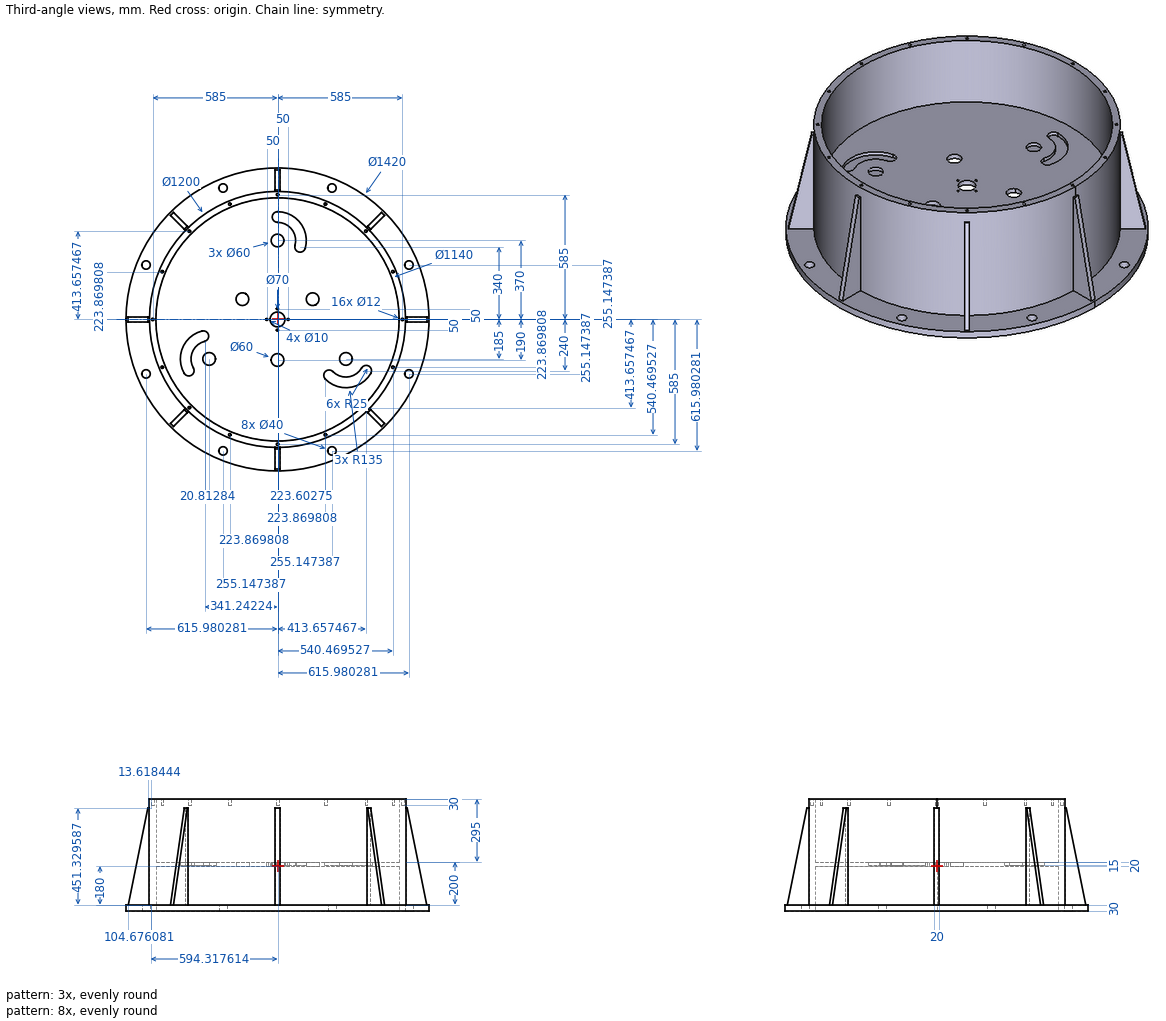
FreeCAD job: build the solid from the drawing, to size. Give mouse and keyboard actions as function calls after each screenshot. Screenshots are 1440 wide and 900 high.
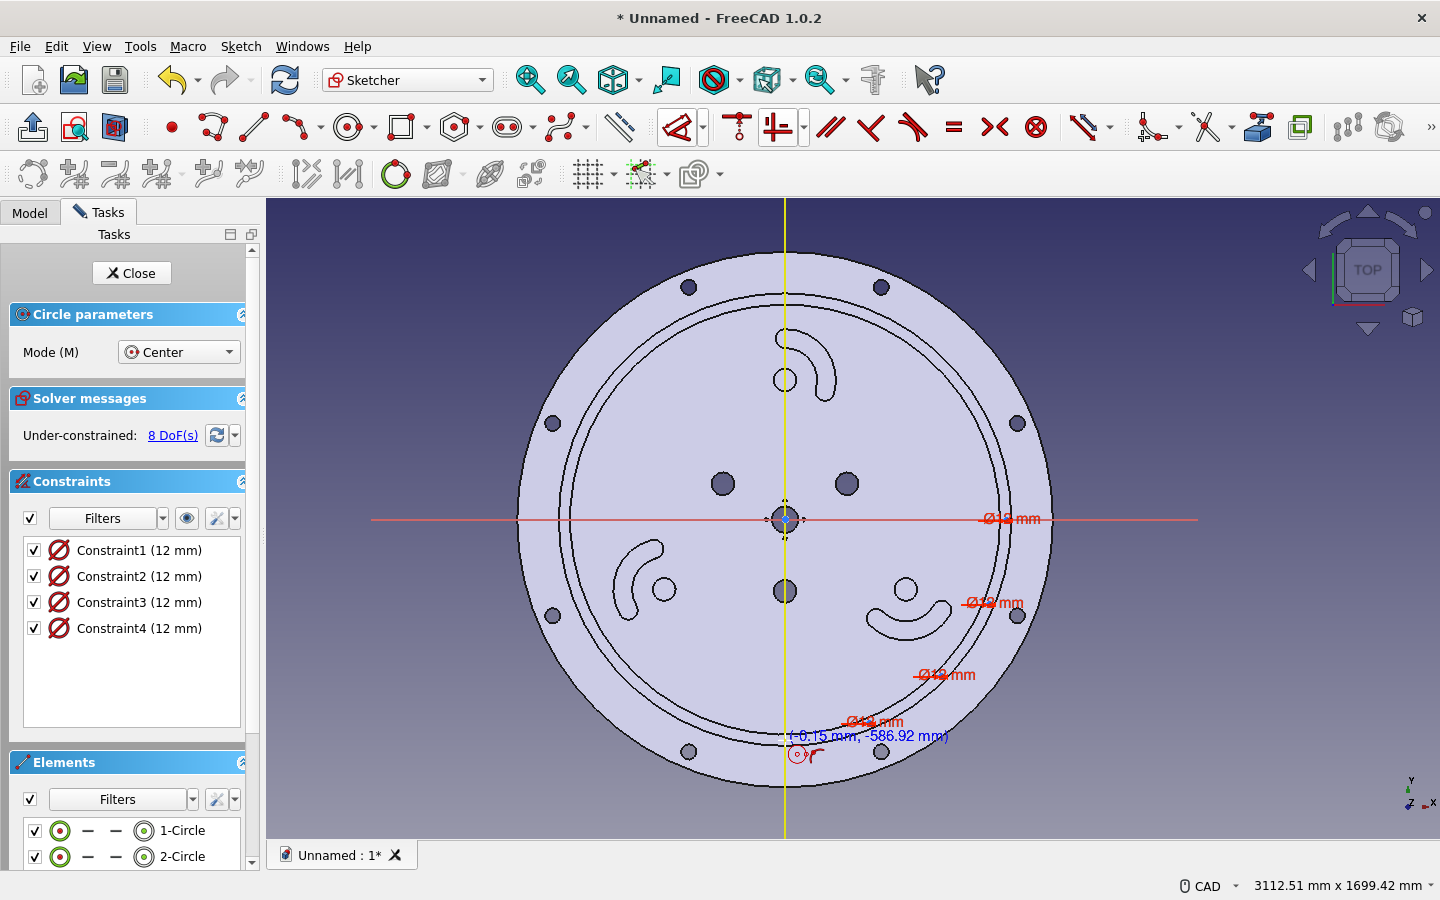
click(785, 740)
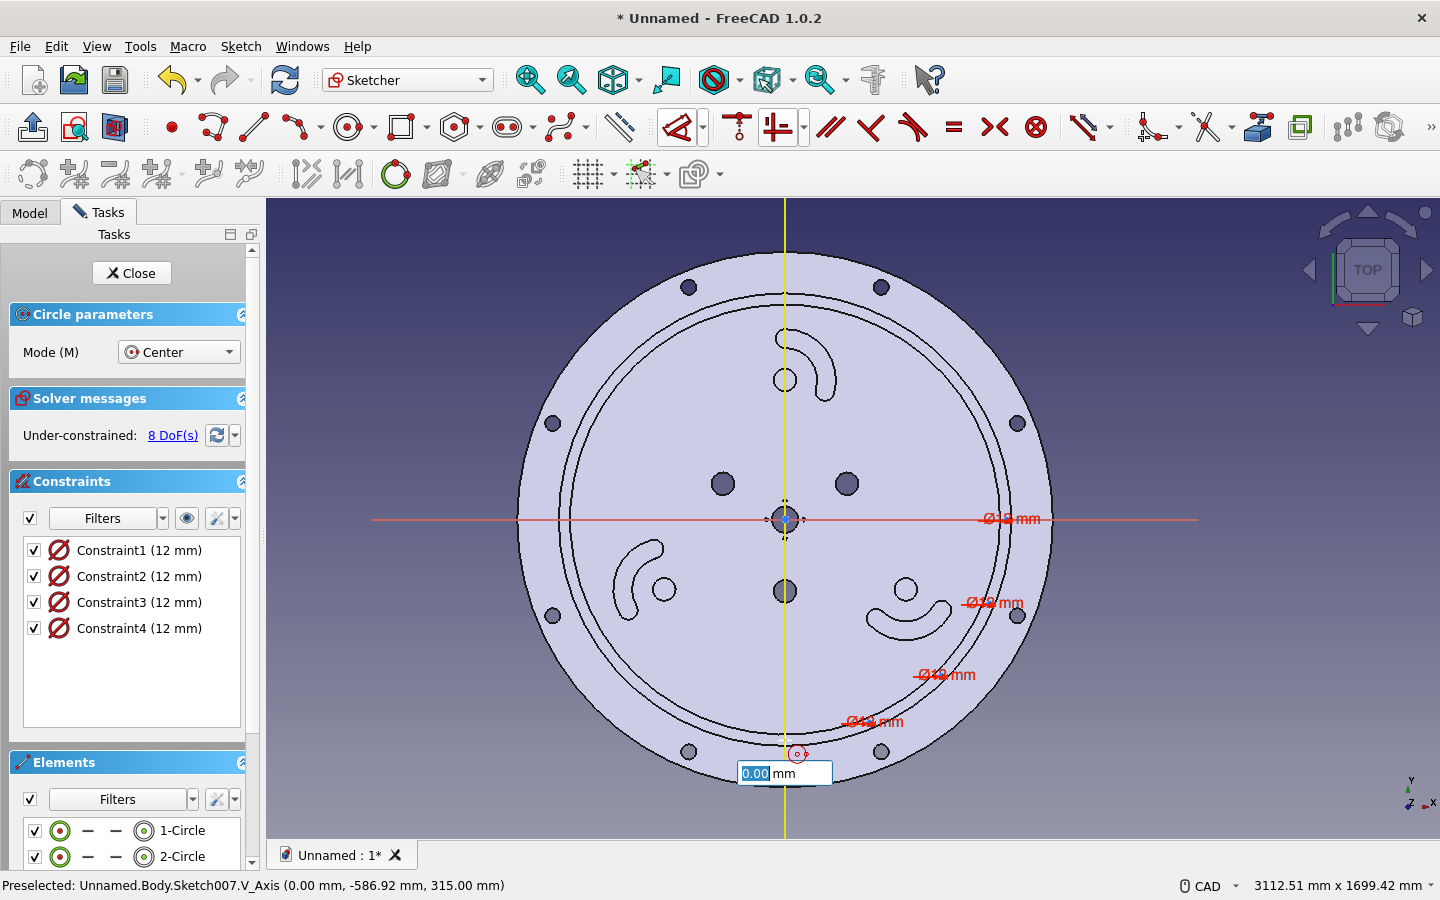
scroll(787, 740, up, 11)
move(785, 729)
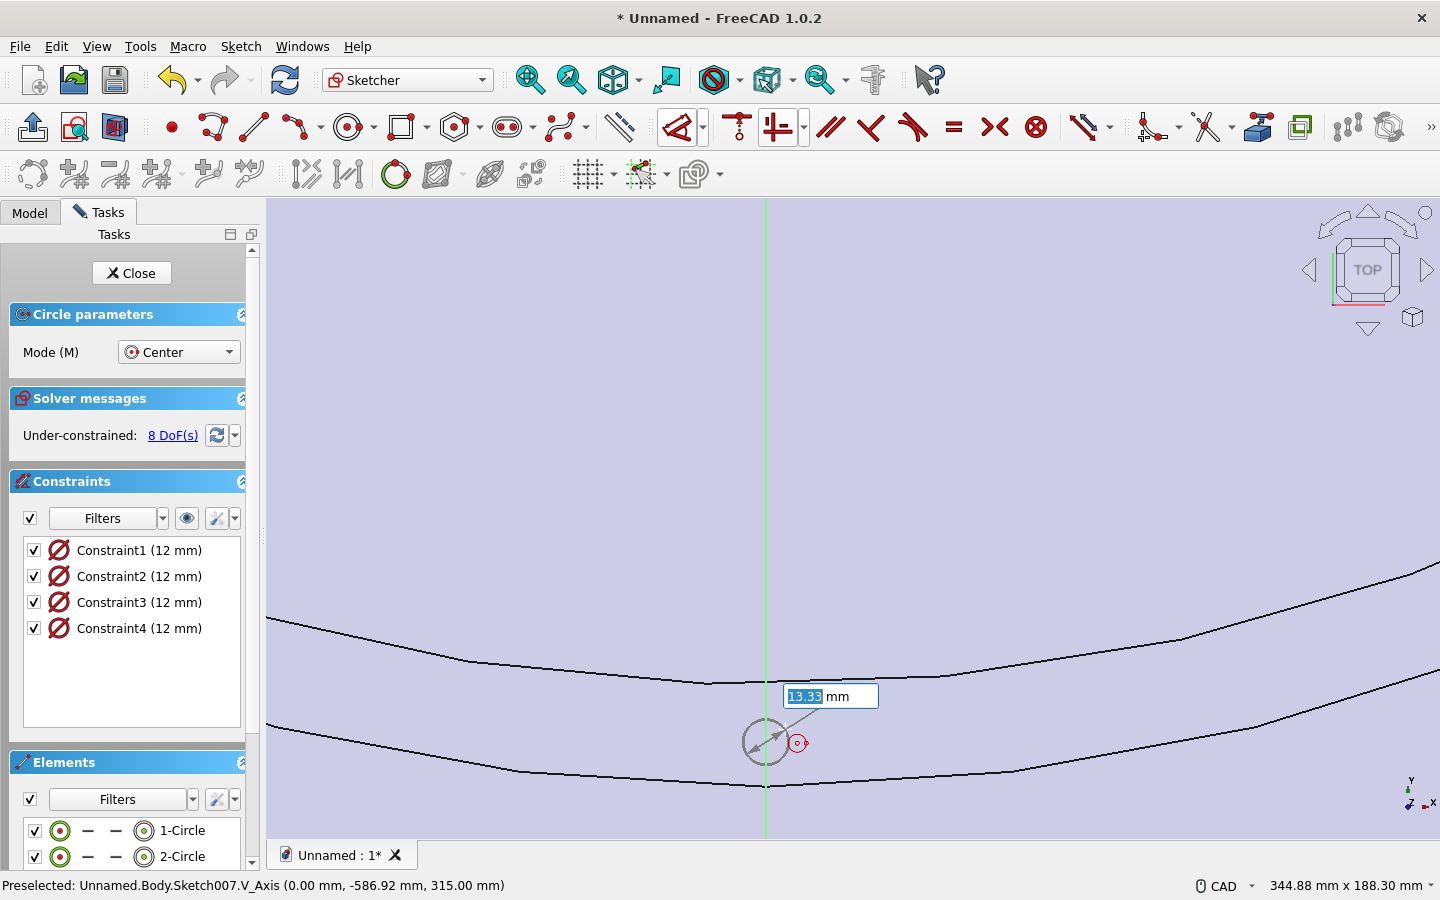
text(12)
key(Return)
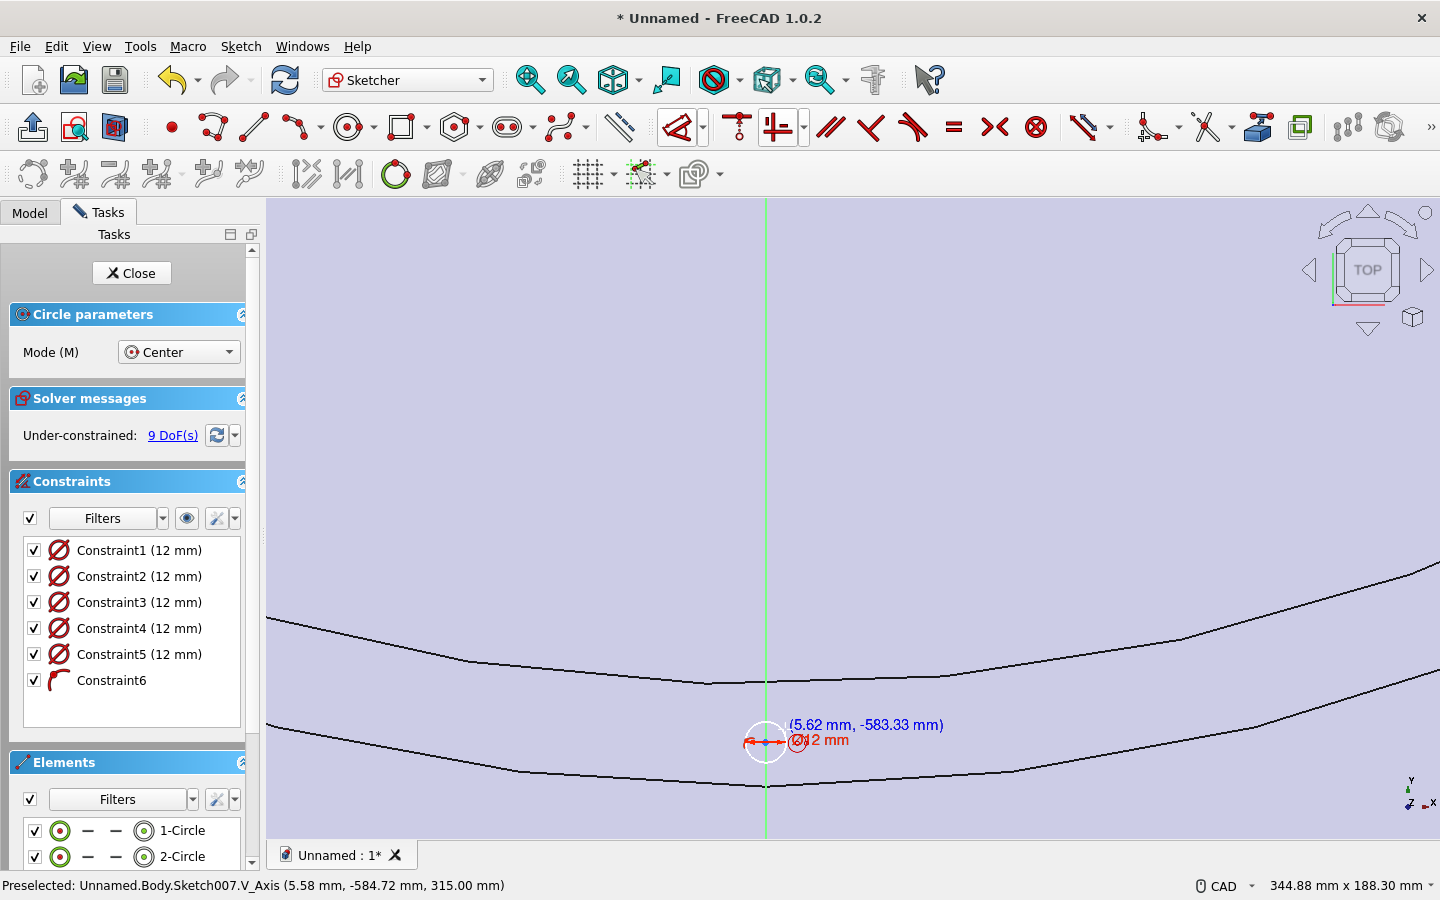
scroll(787, 740, down, 11)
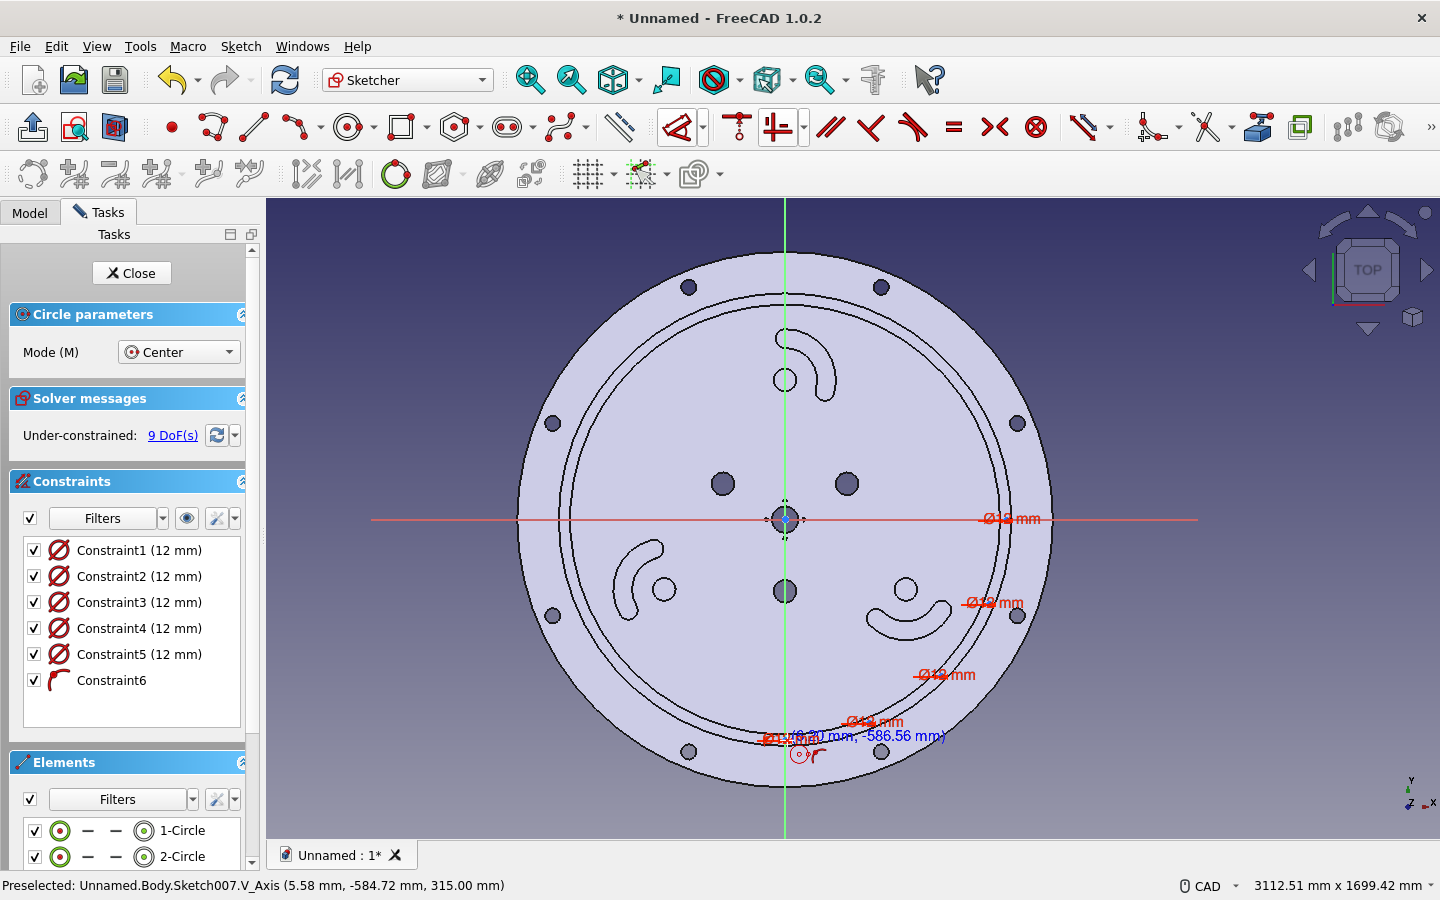
scroll(701, 723, up, 12)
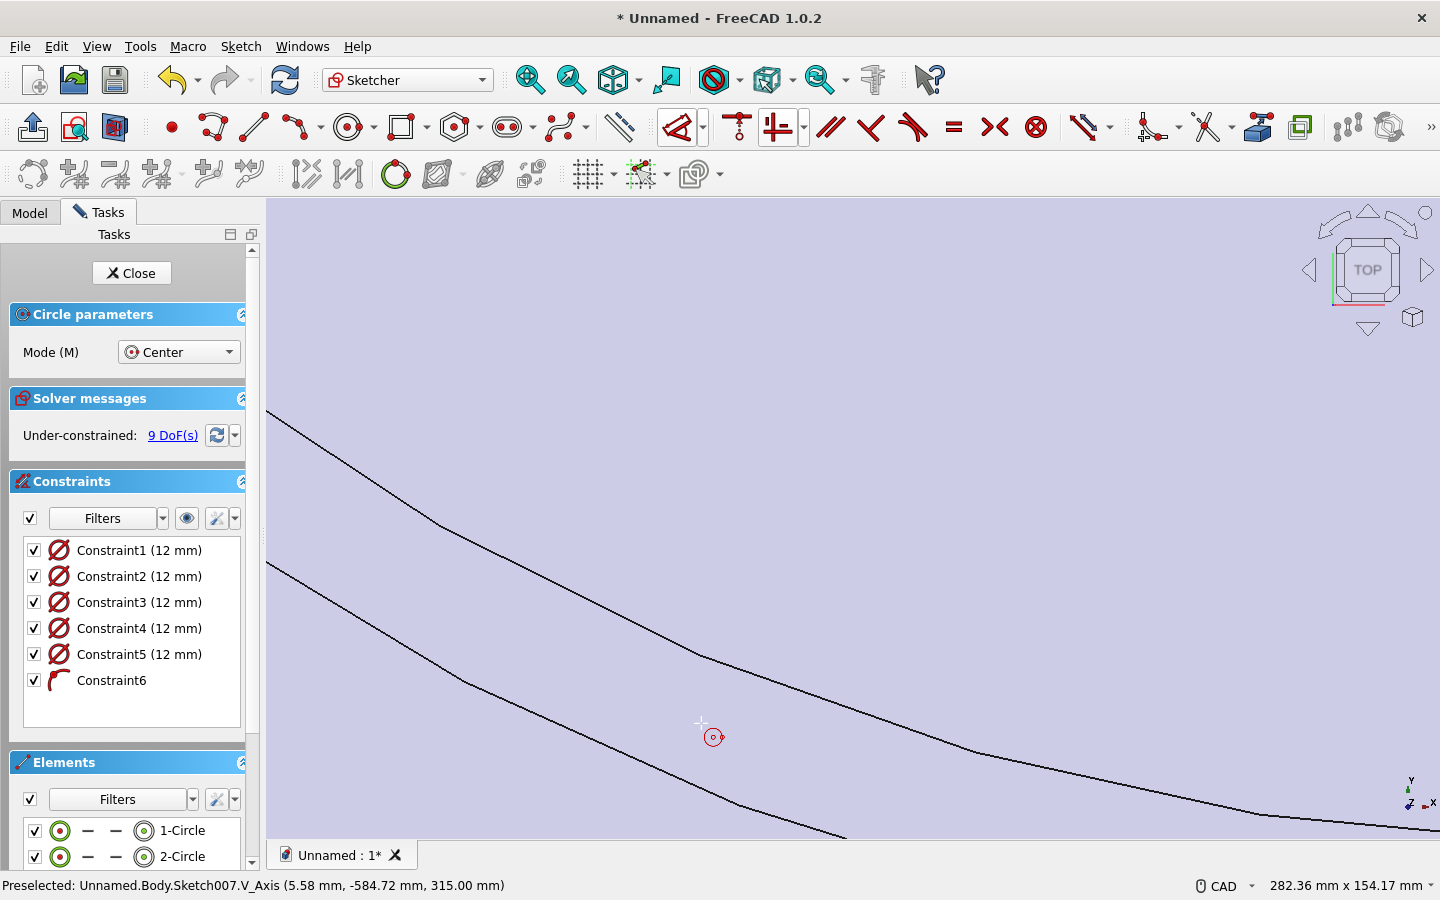
scroll(701, 723, down, 12)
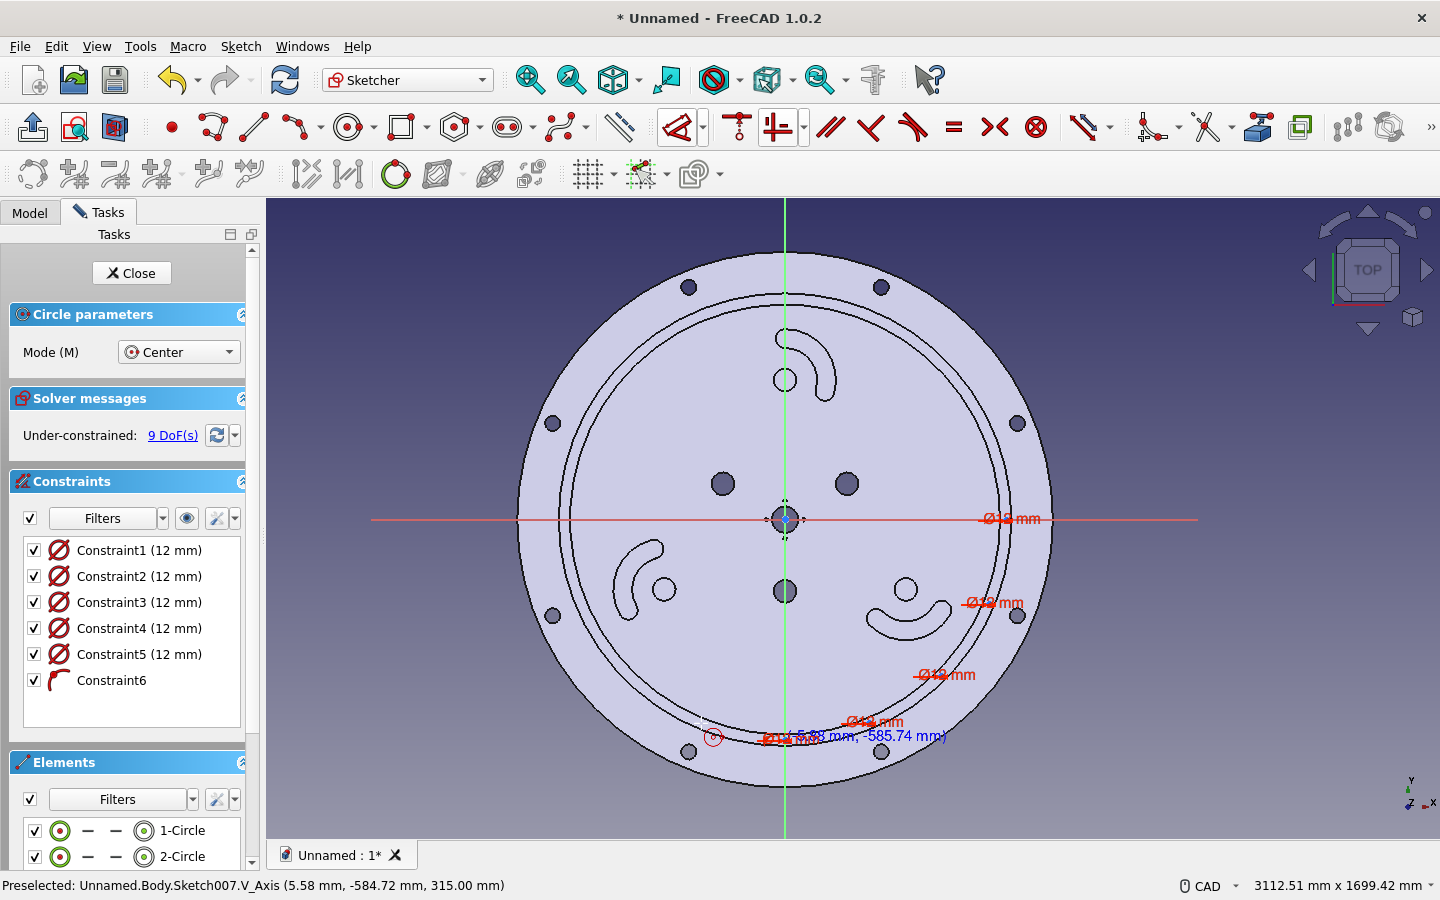
click(701, 723)
move(702, 722)